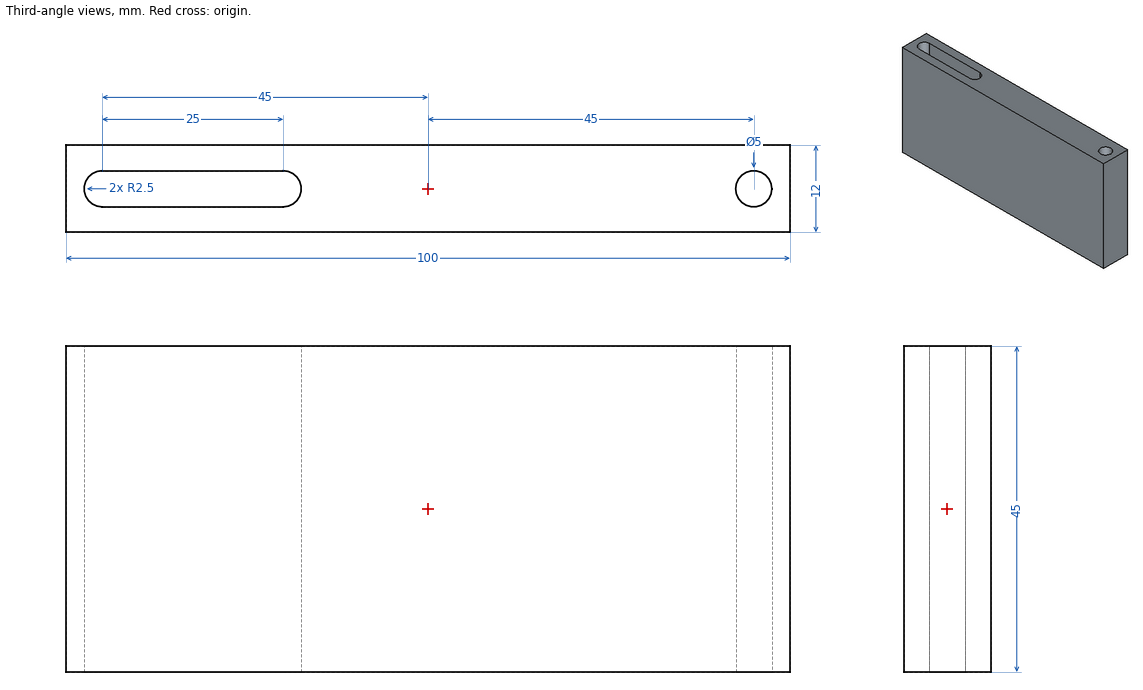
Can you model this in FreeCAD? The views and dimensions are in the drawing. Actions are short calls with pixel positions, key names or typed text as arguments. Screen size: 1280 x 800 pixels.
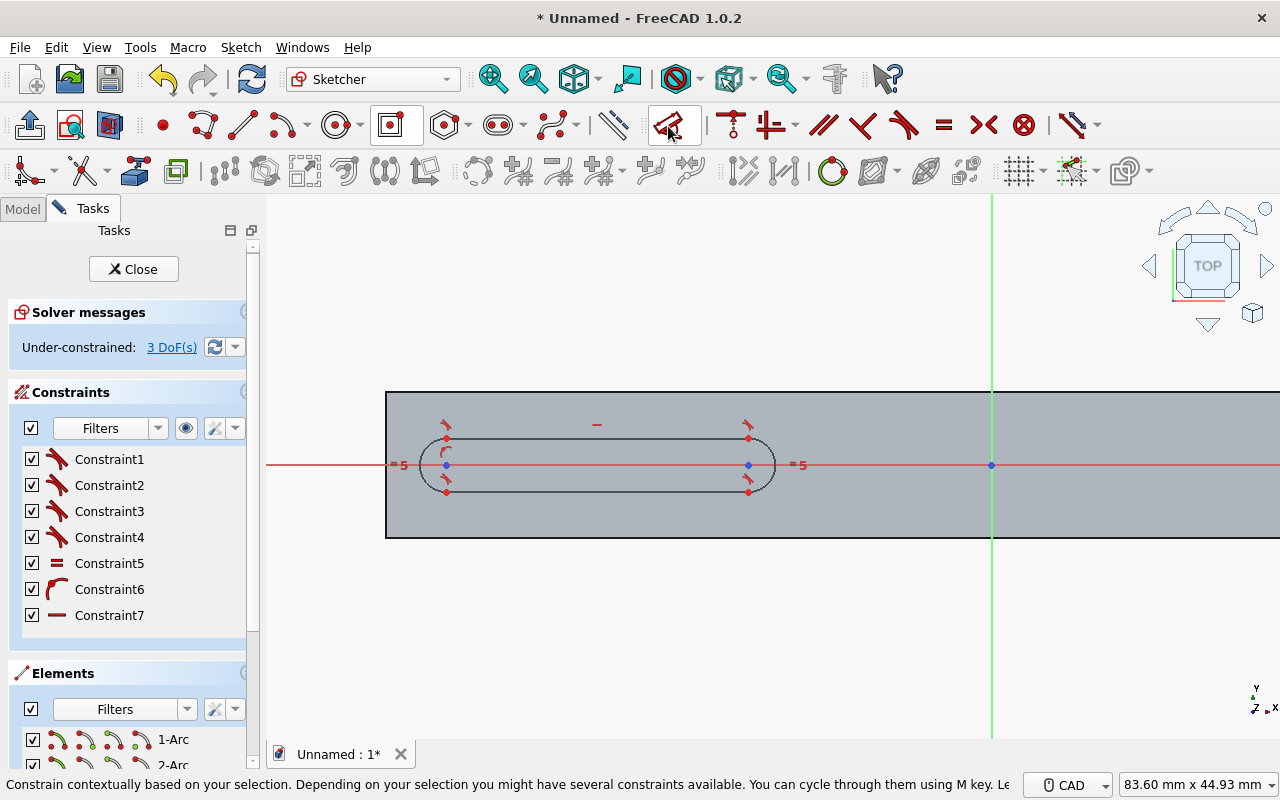
scroll(425, 450, up, 2)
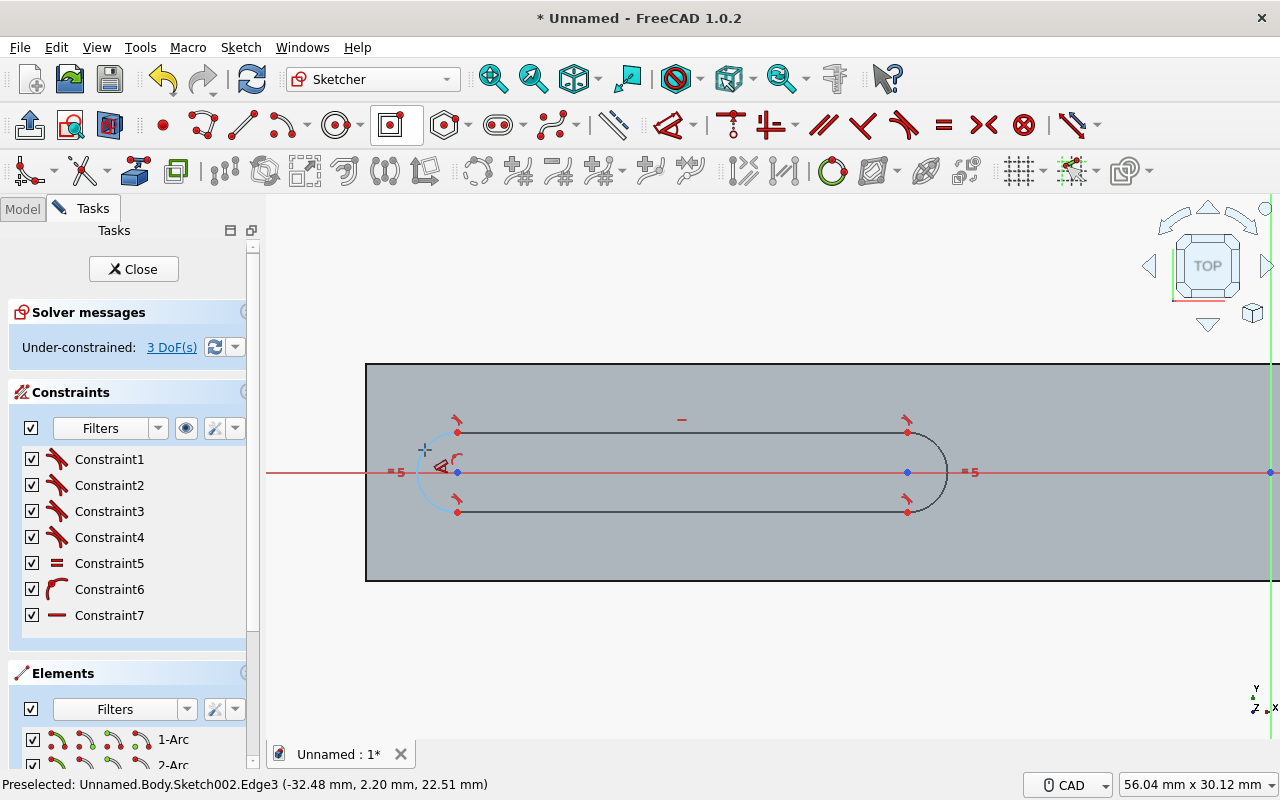
click(425, 449)
click(399, 430)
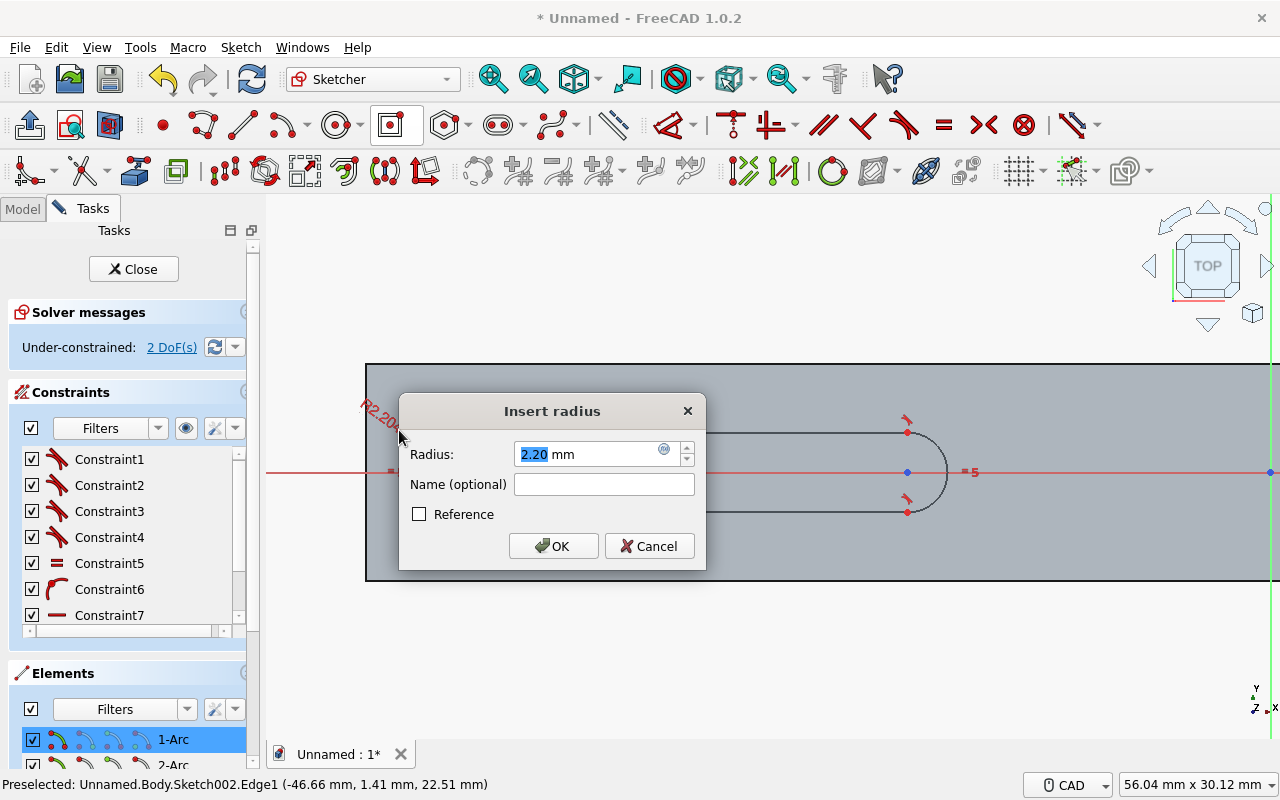
text(2.5)
key(Return)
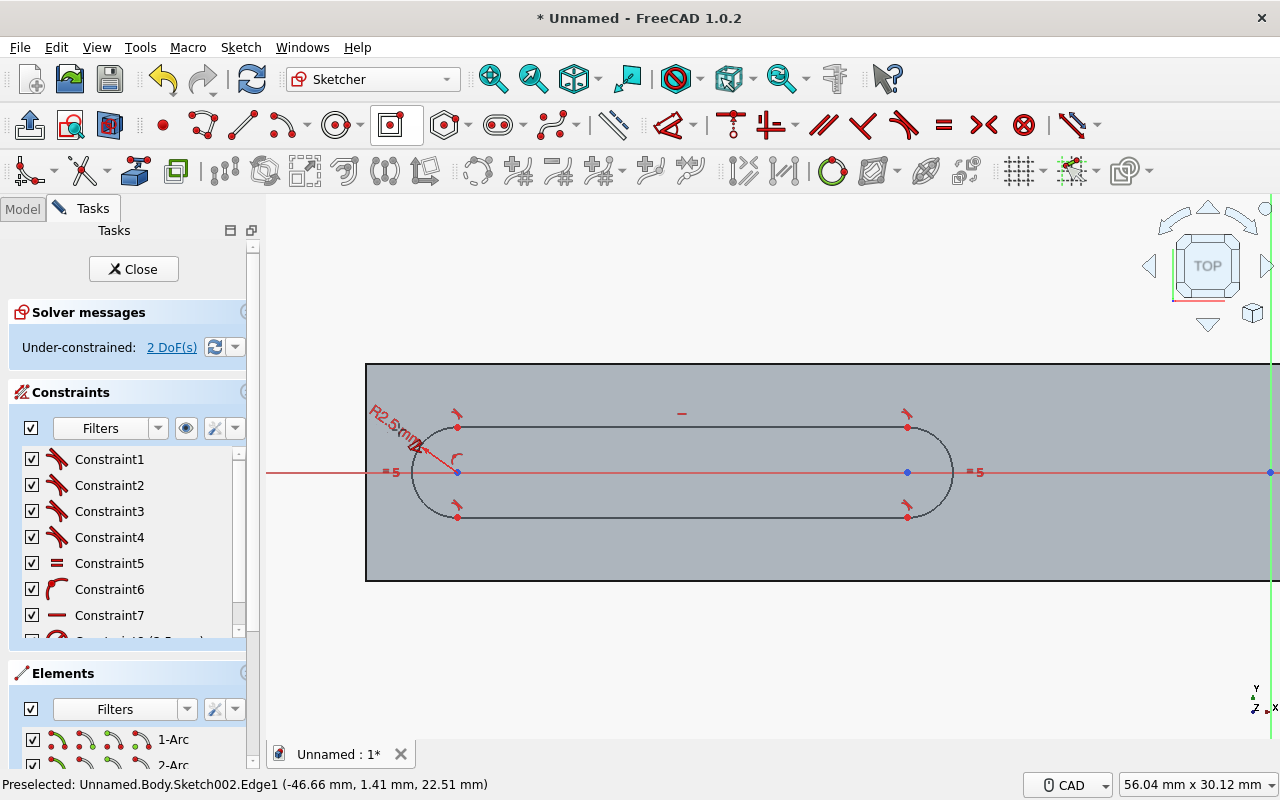
click(592, 427)
click(682, 393)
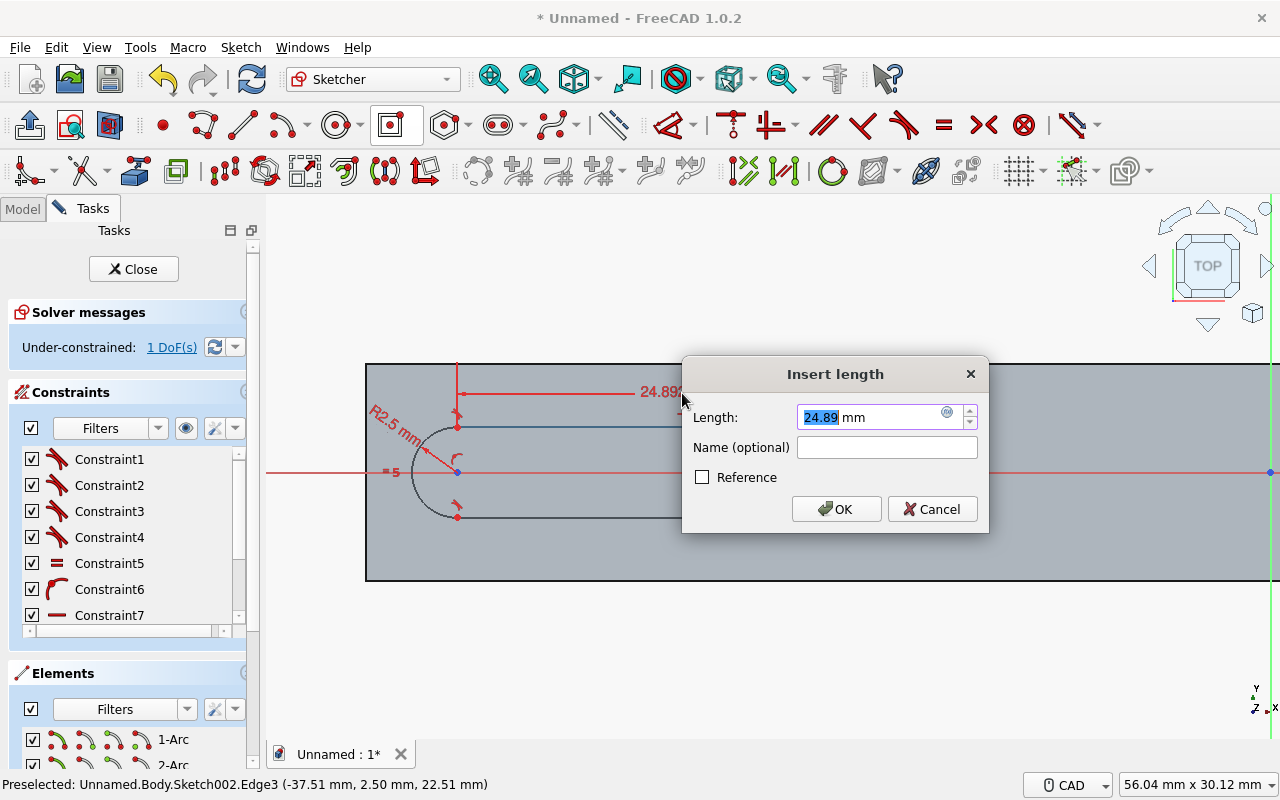
text(25)
key(Return)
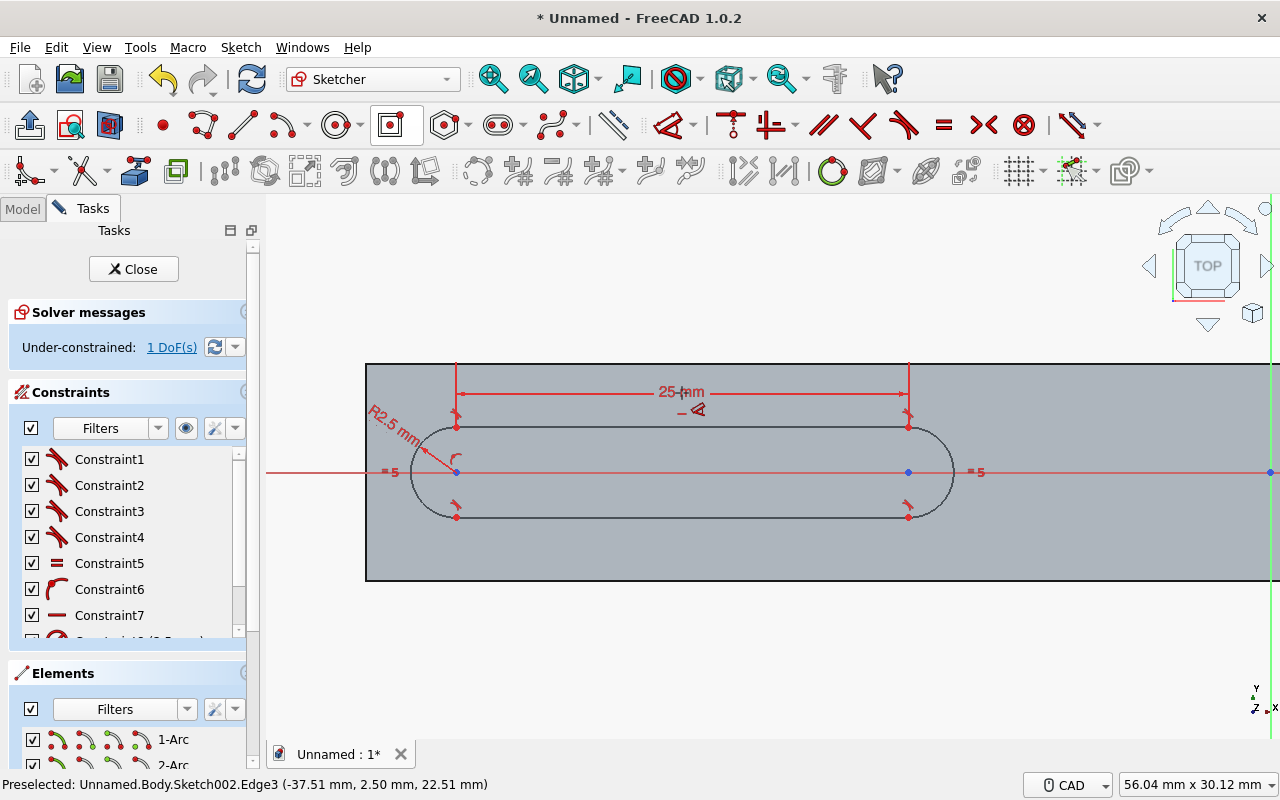
click(456, 427)
click(786, 393)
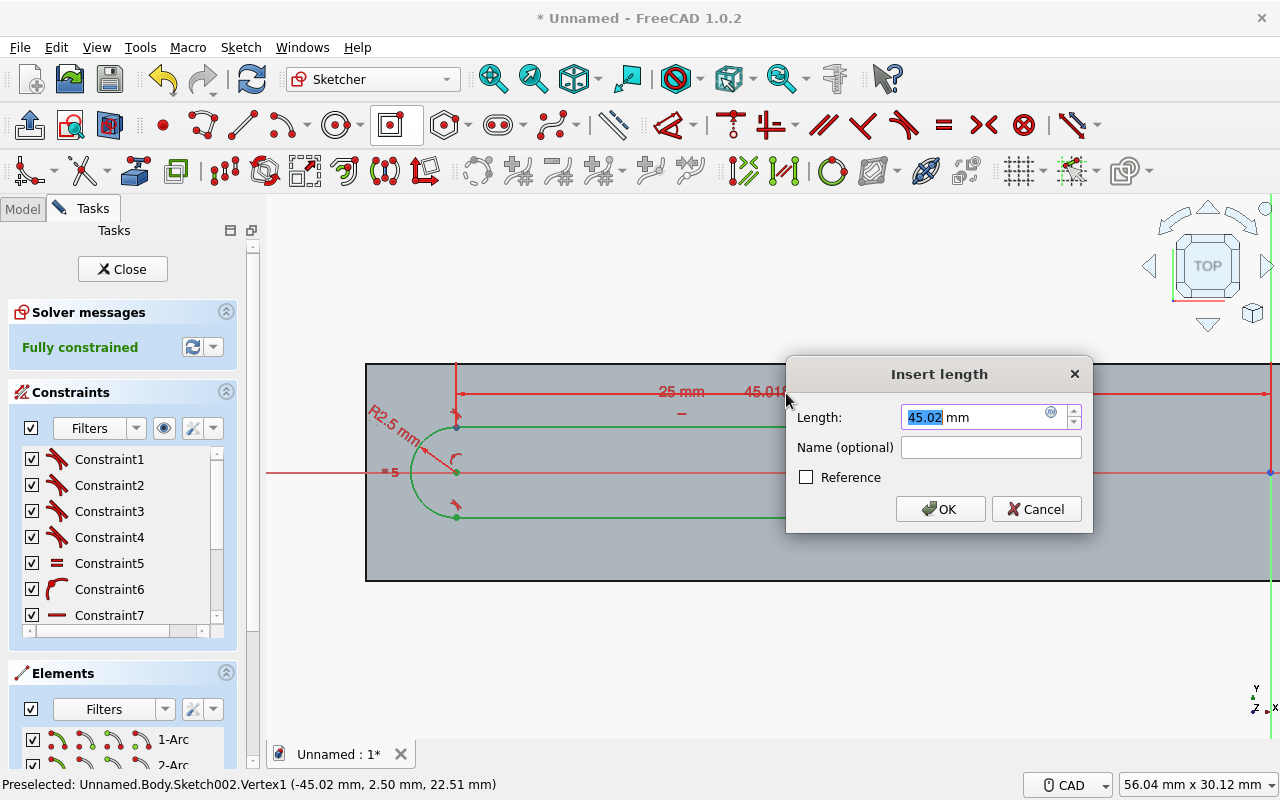
text(45)
key(Return)
key(Escape)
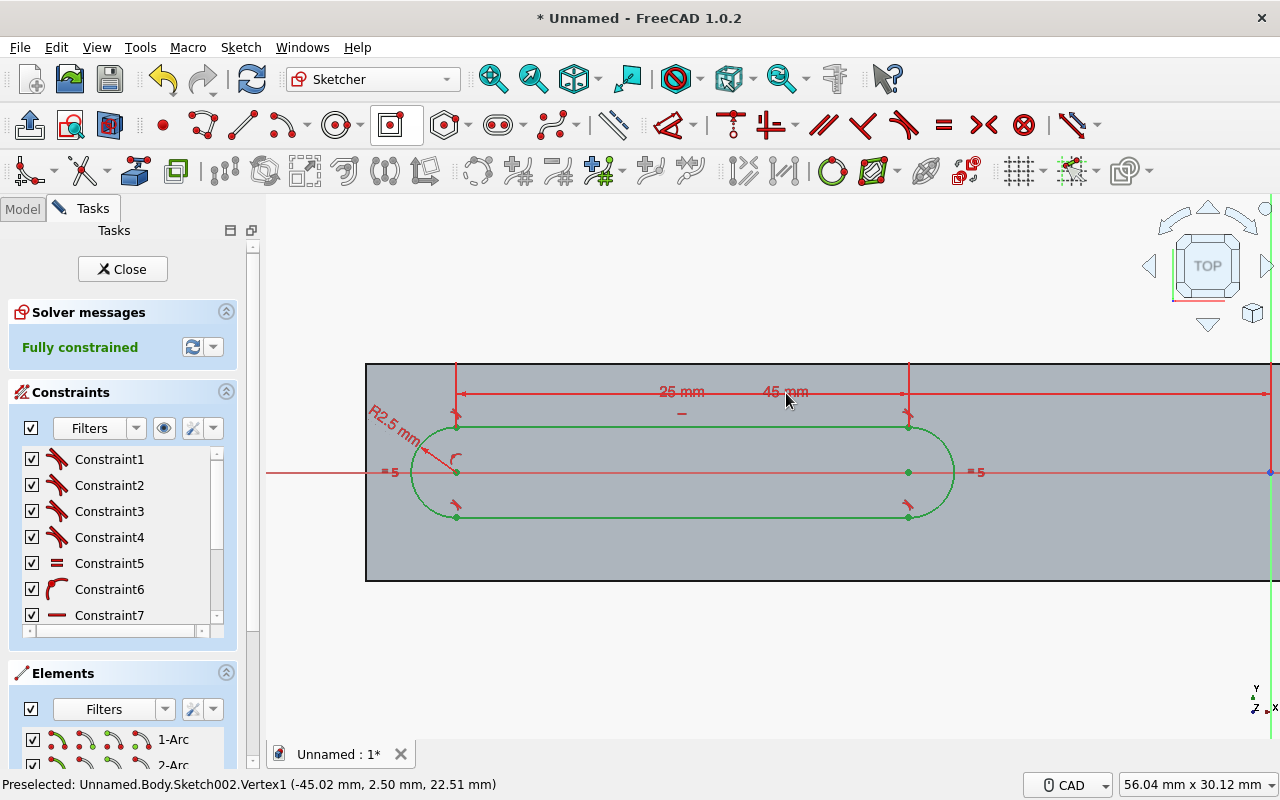
click(123, 269)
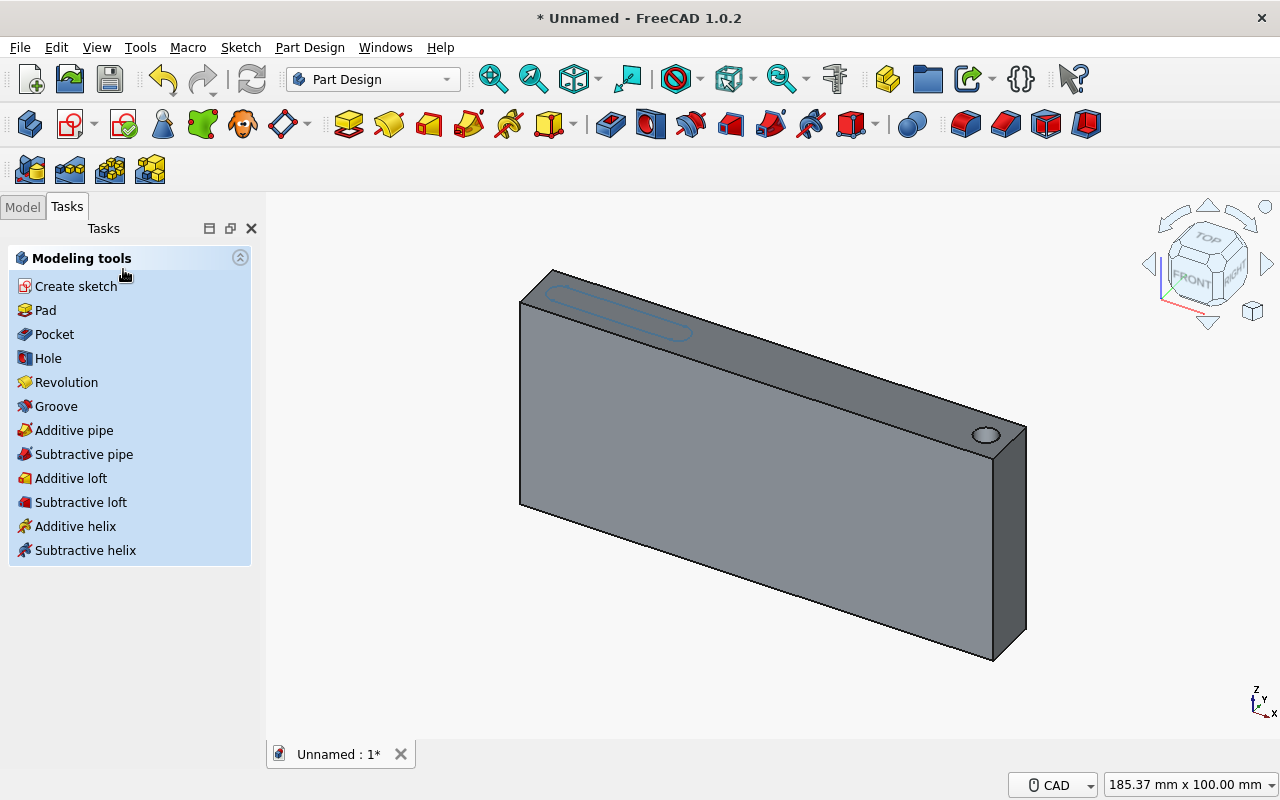
click(612, 124)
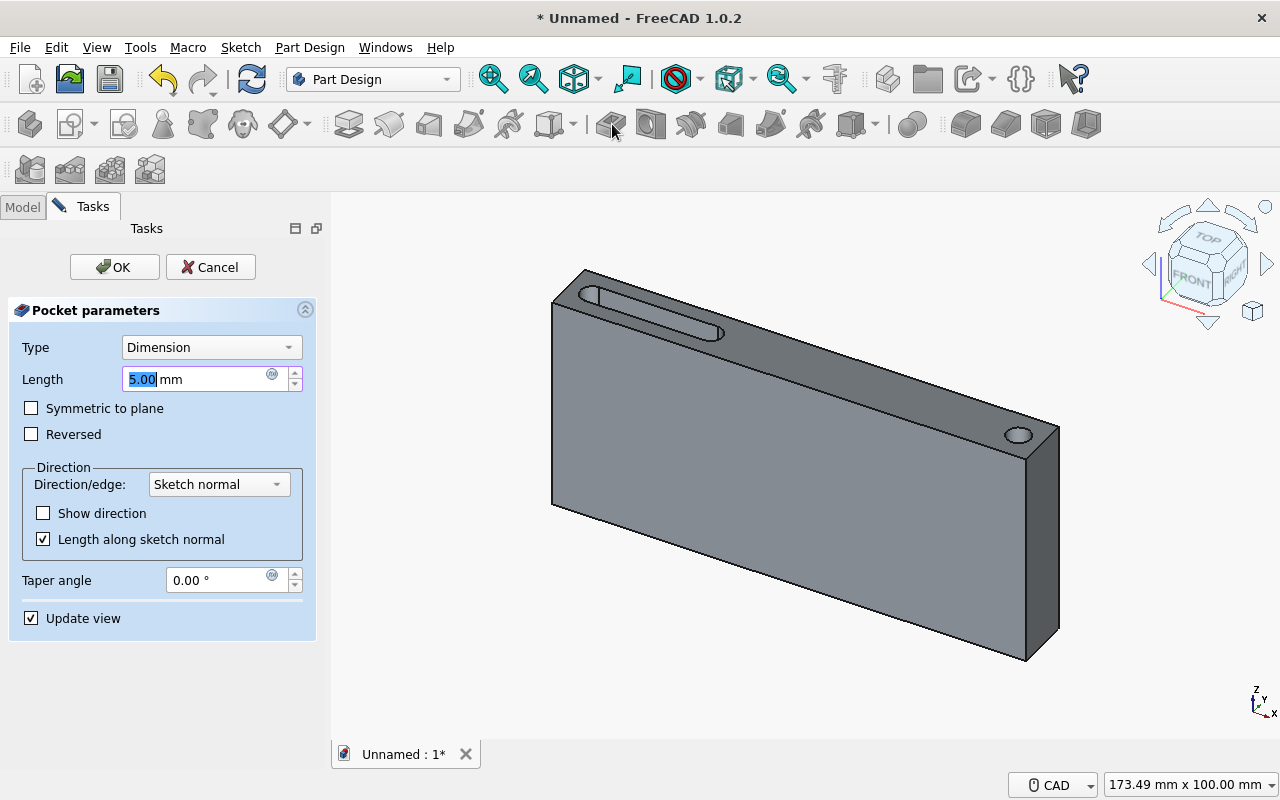
click(212, 348)